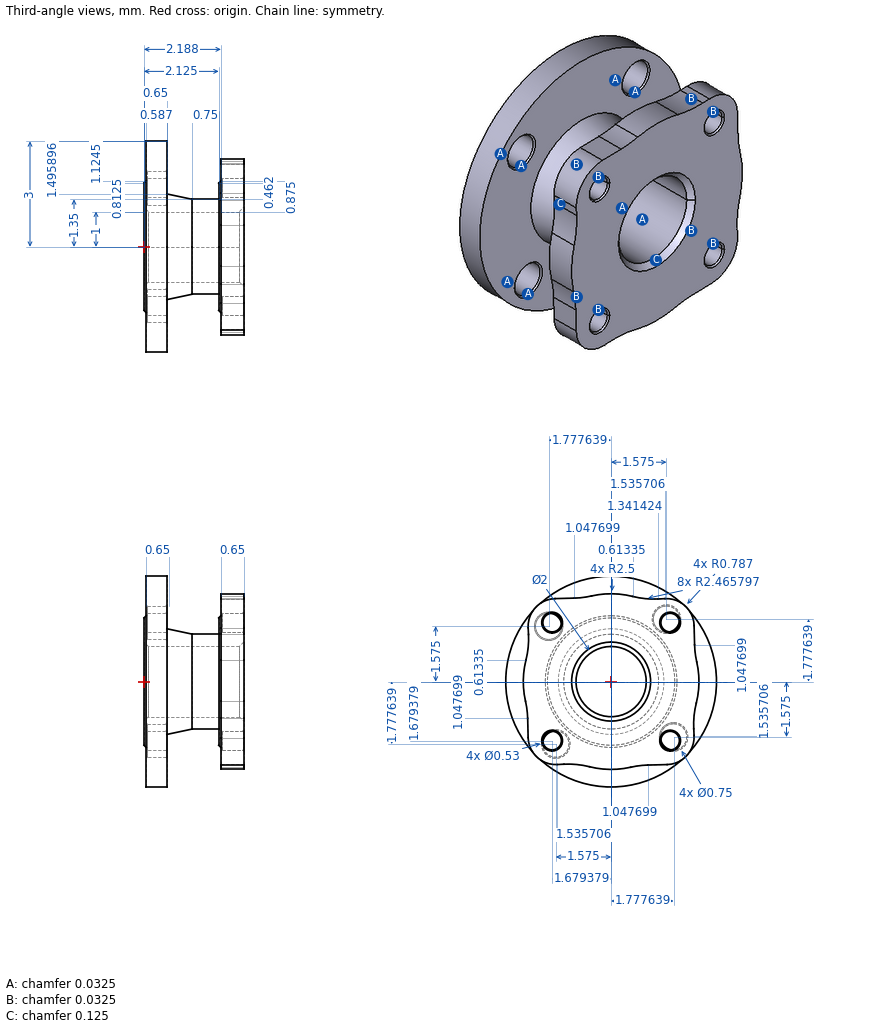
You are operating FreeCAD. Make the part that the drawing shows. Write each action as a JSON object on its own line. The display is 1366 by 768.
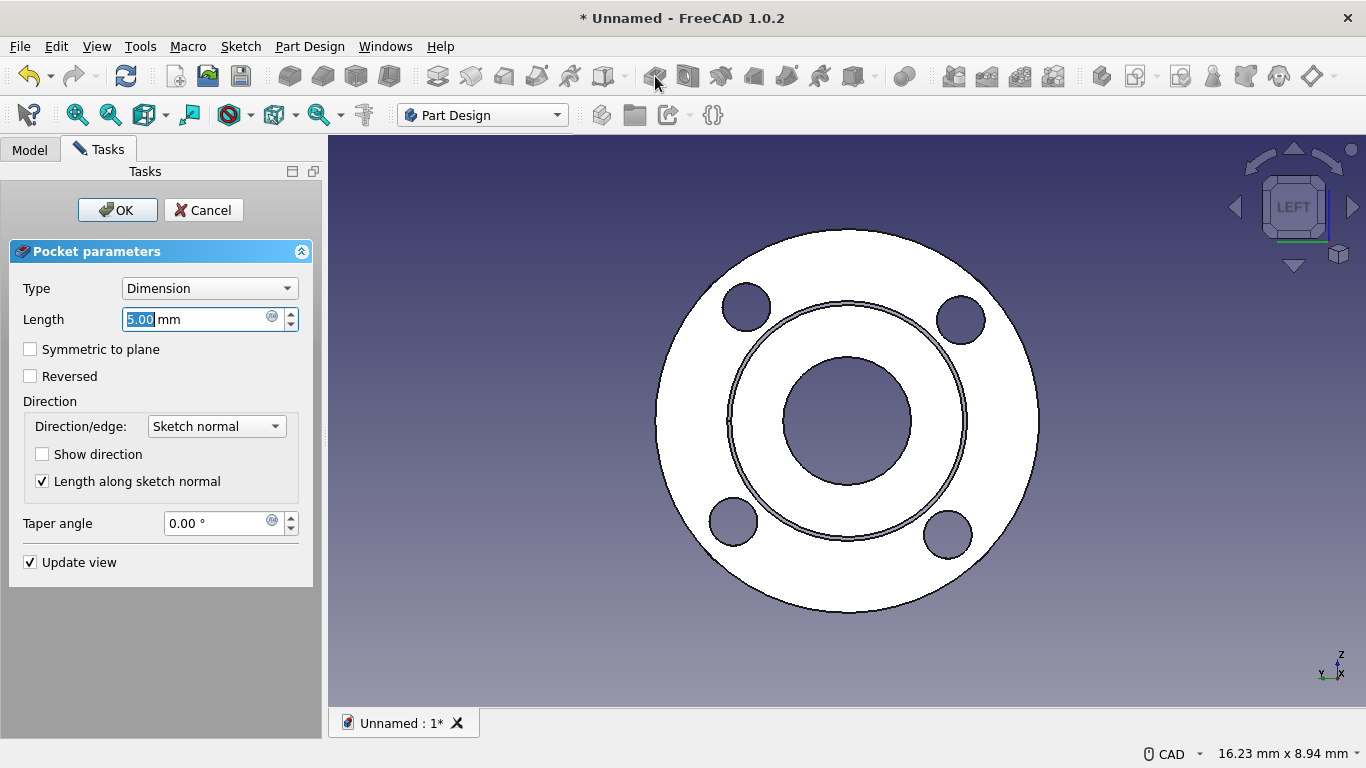
{"action": "type", "text": "0.65"}
{"action": "key", "text": "Tab"}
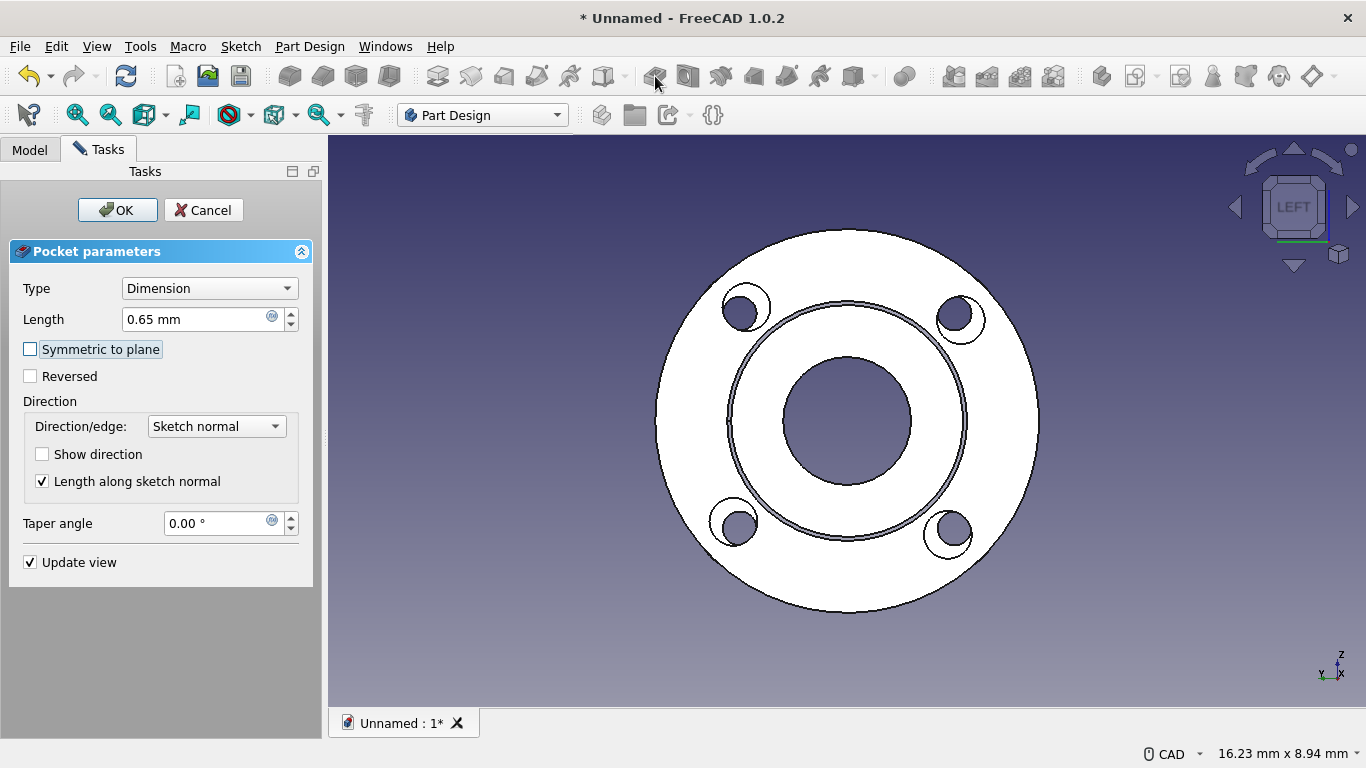
{"action": "left_click", "coordinate": [118, 210]}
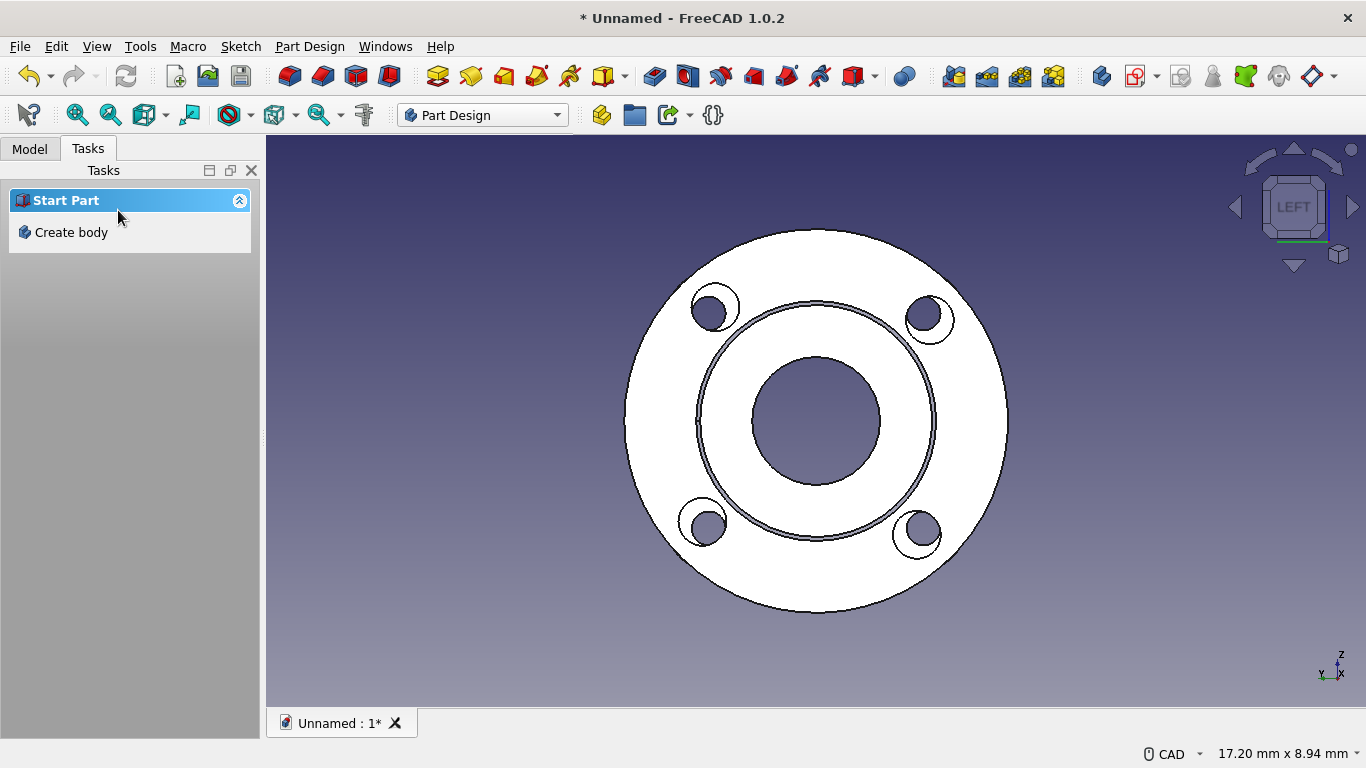
{"action": "left_click", "coordinate": [906, 319]}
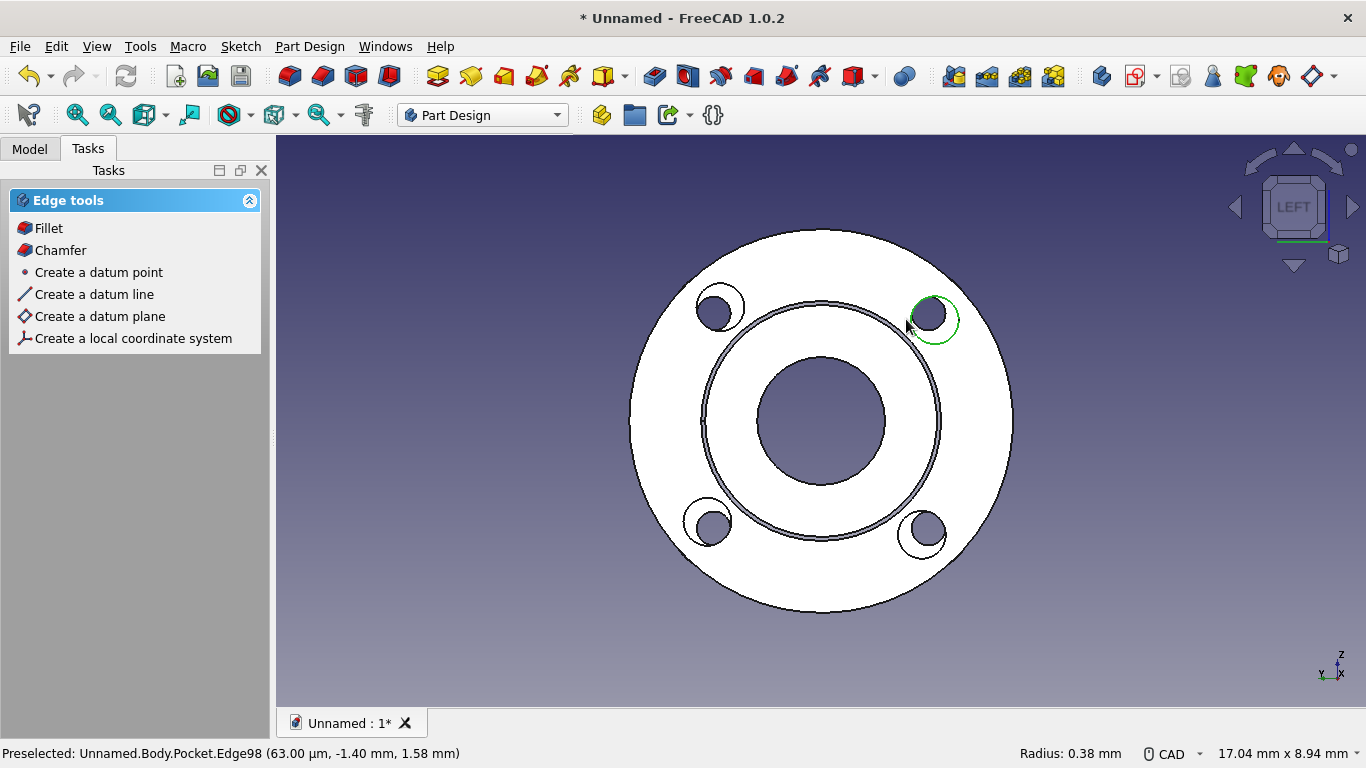
{"action": "left_click", "coordinate": [696, 306], "text": "ctrl"}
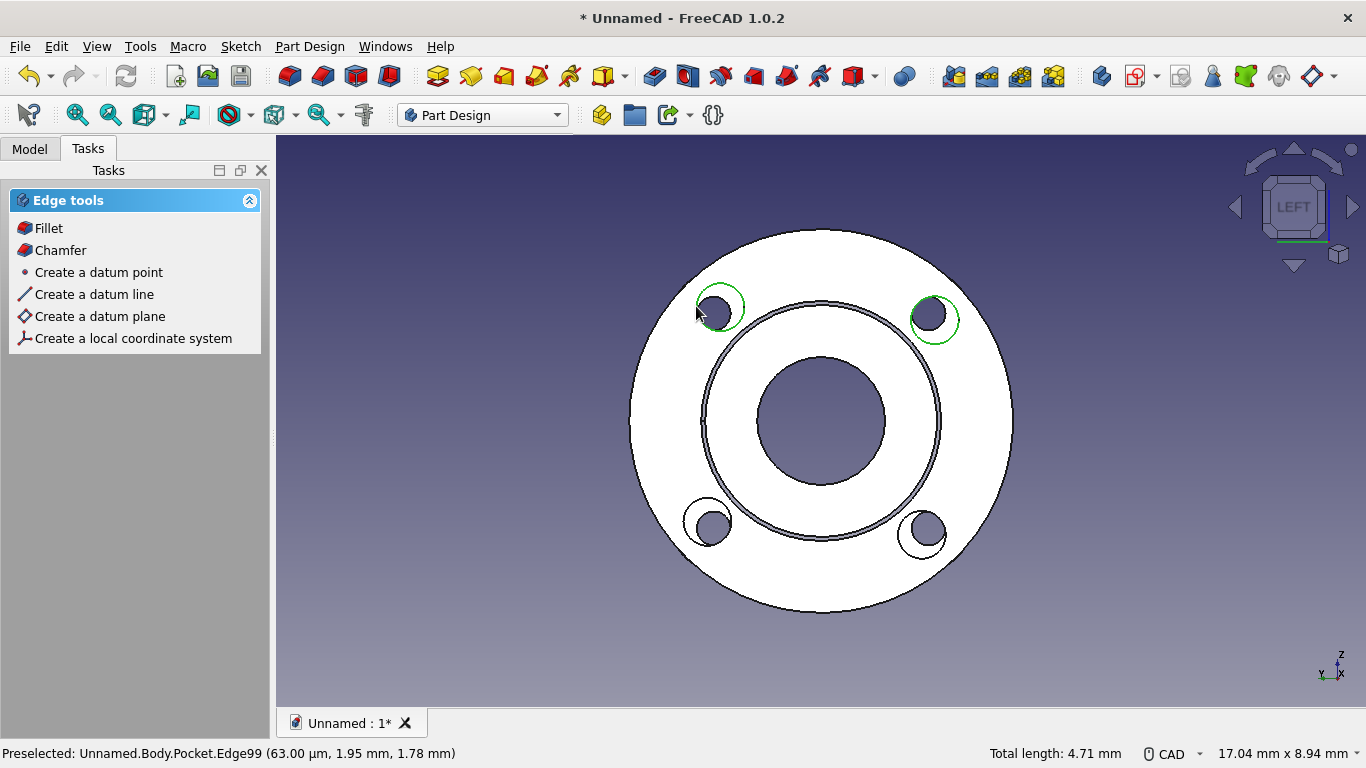
{"action": "left_click", "coordinate": [683, 521], "text": "ctrl"}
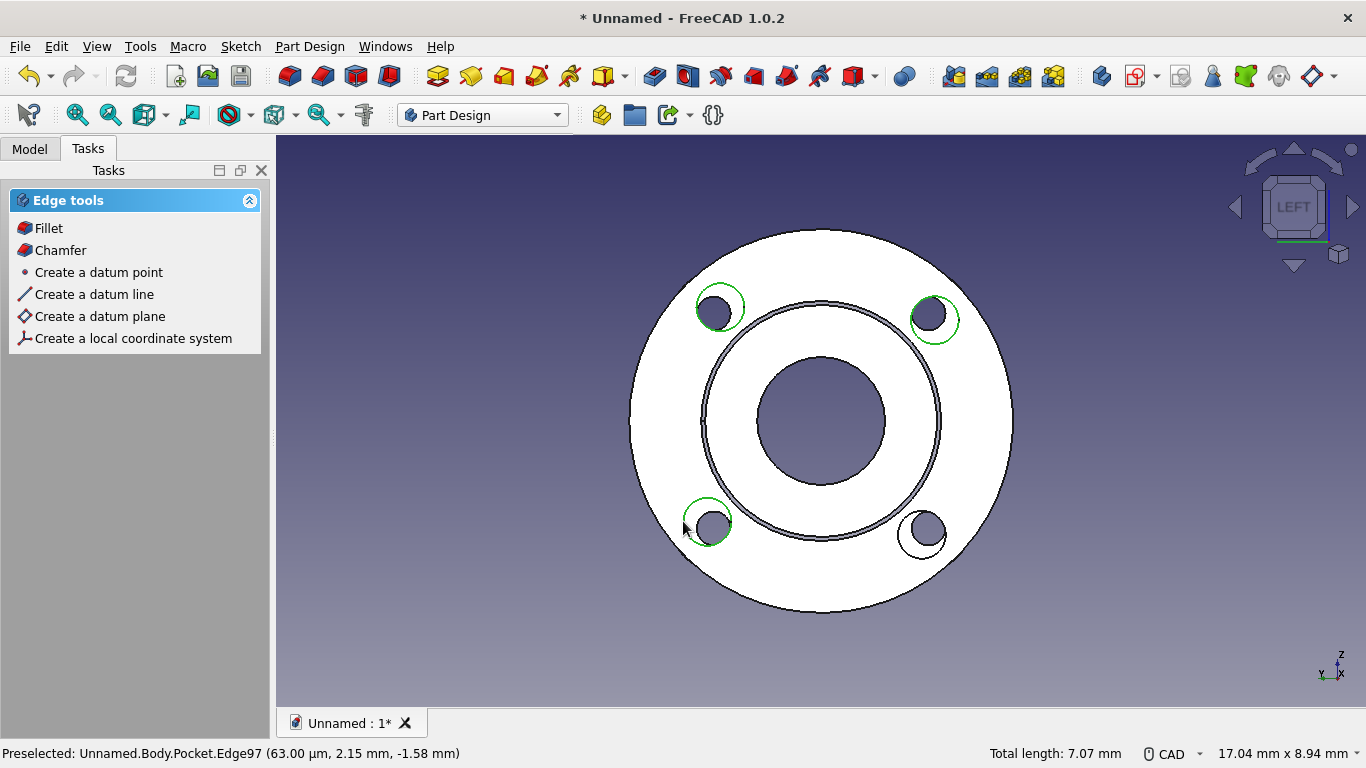
{"action": "left_click", "coordinate": [898, 534], "text": "ctrl"}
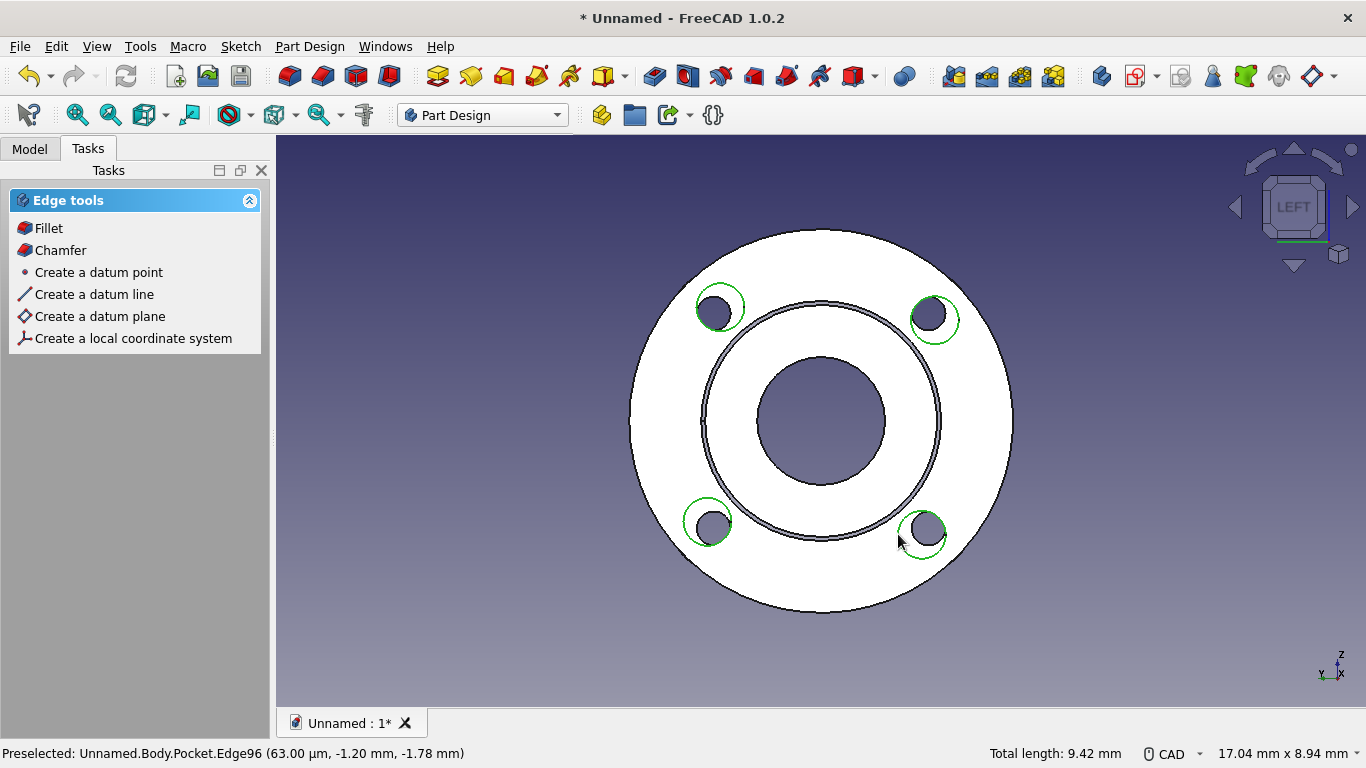
{"action": "key", "text": "0"}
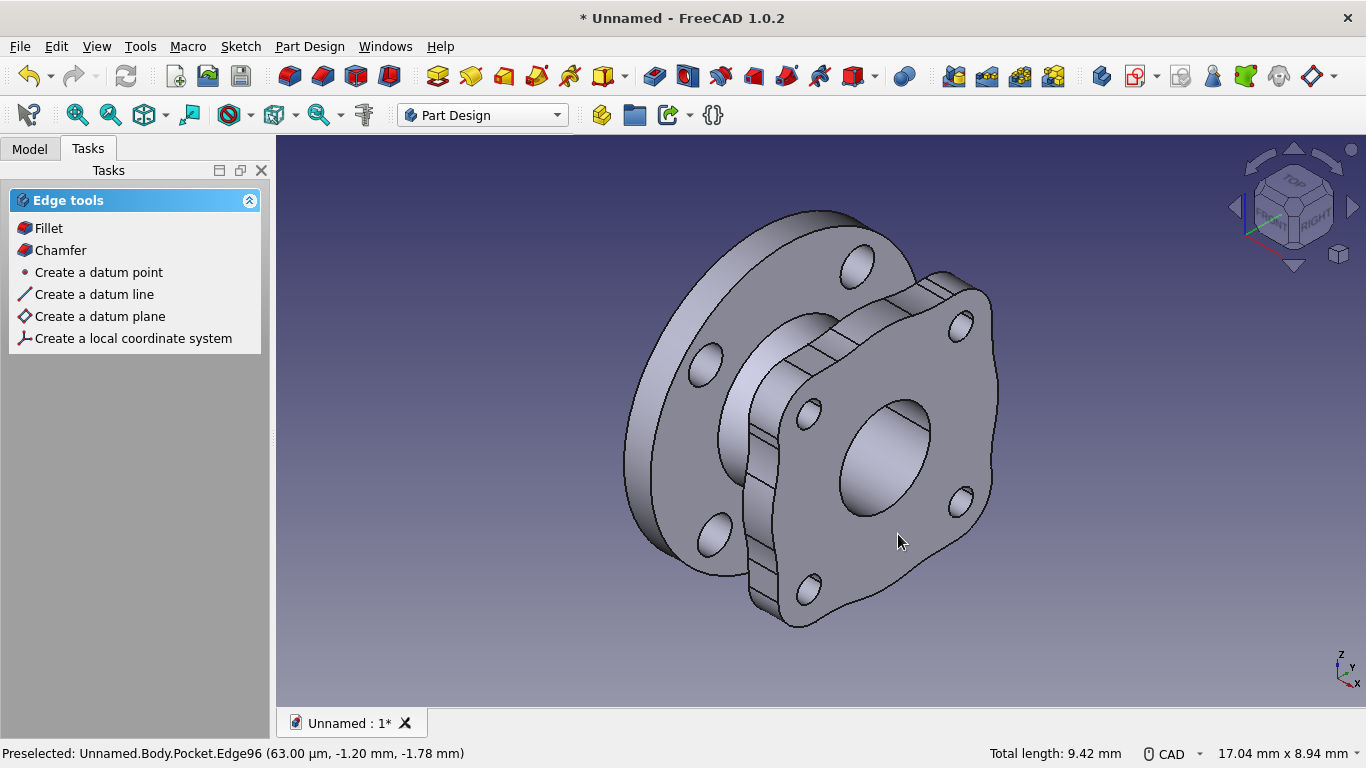
{"action": "left_click", "coordinate": [723, 354], "text": "ctrl"}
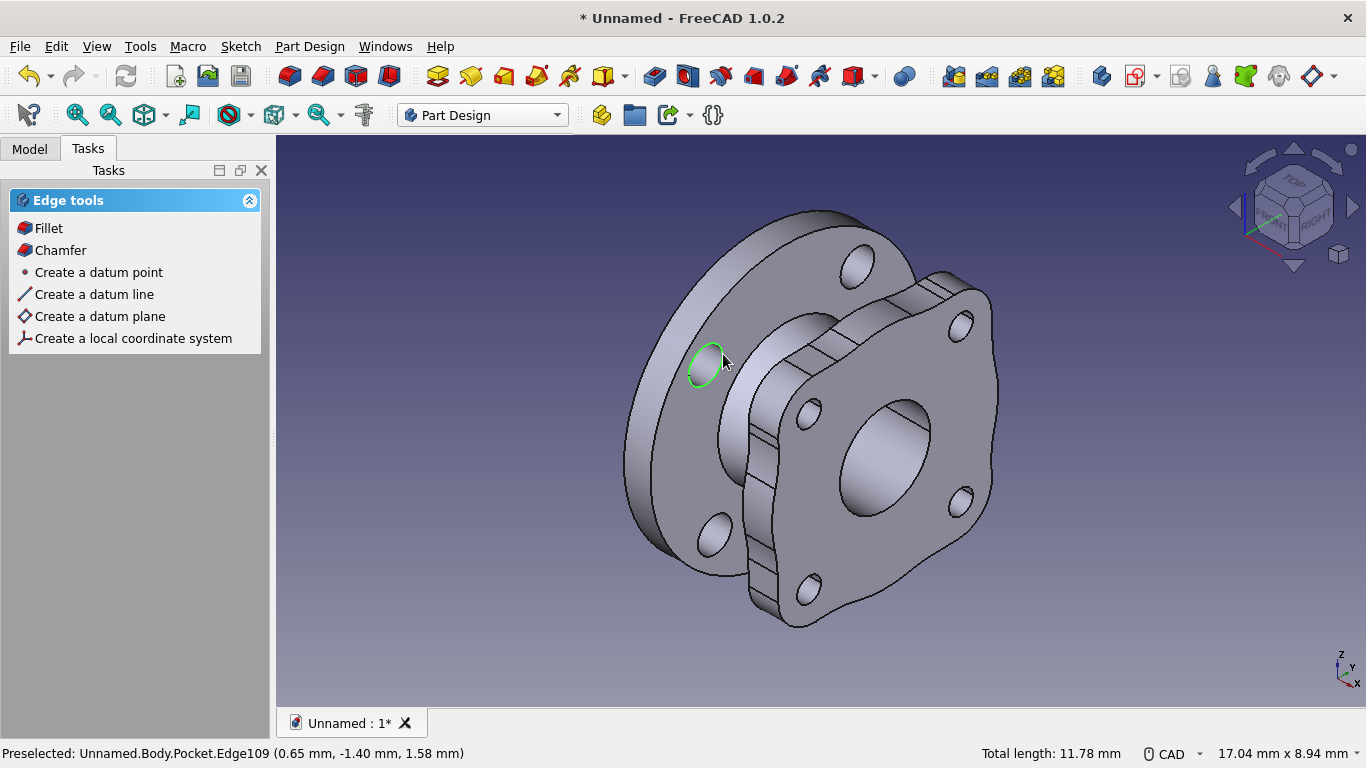
{"action": "left_click", "coordinate": [874, 256], "text": "ctrl"}